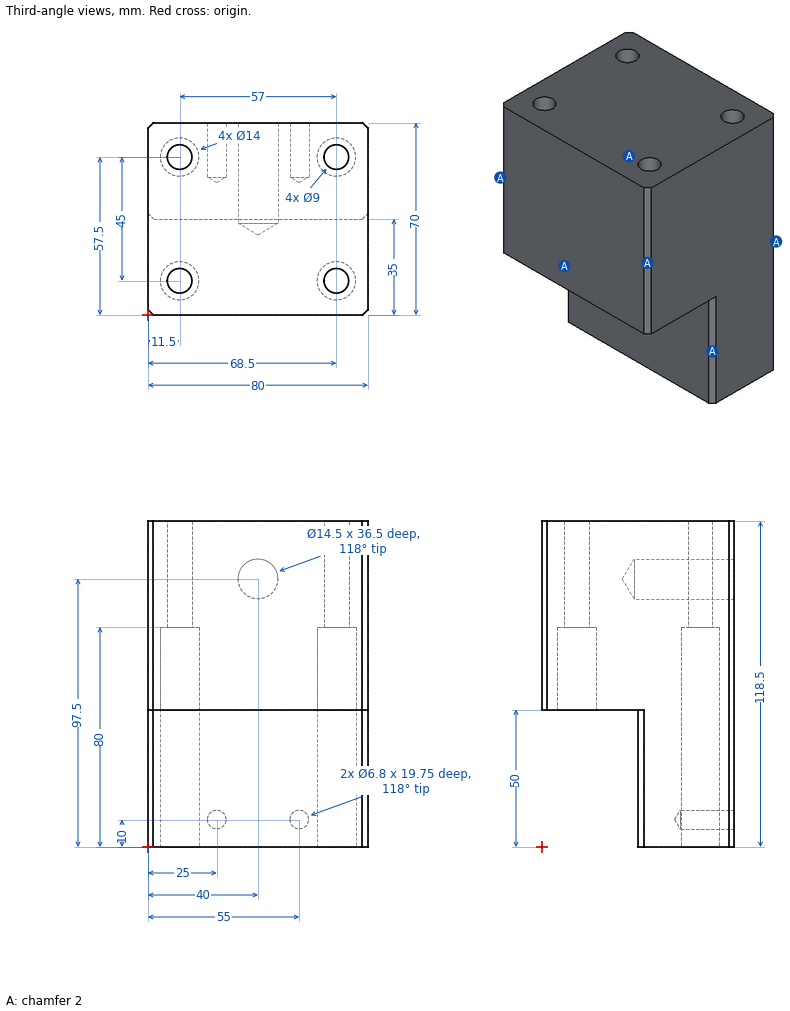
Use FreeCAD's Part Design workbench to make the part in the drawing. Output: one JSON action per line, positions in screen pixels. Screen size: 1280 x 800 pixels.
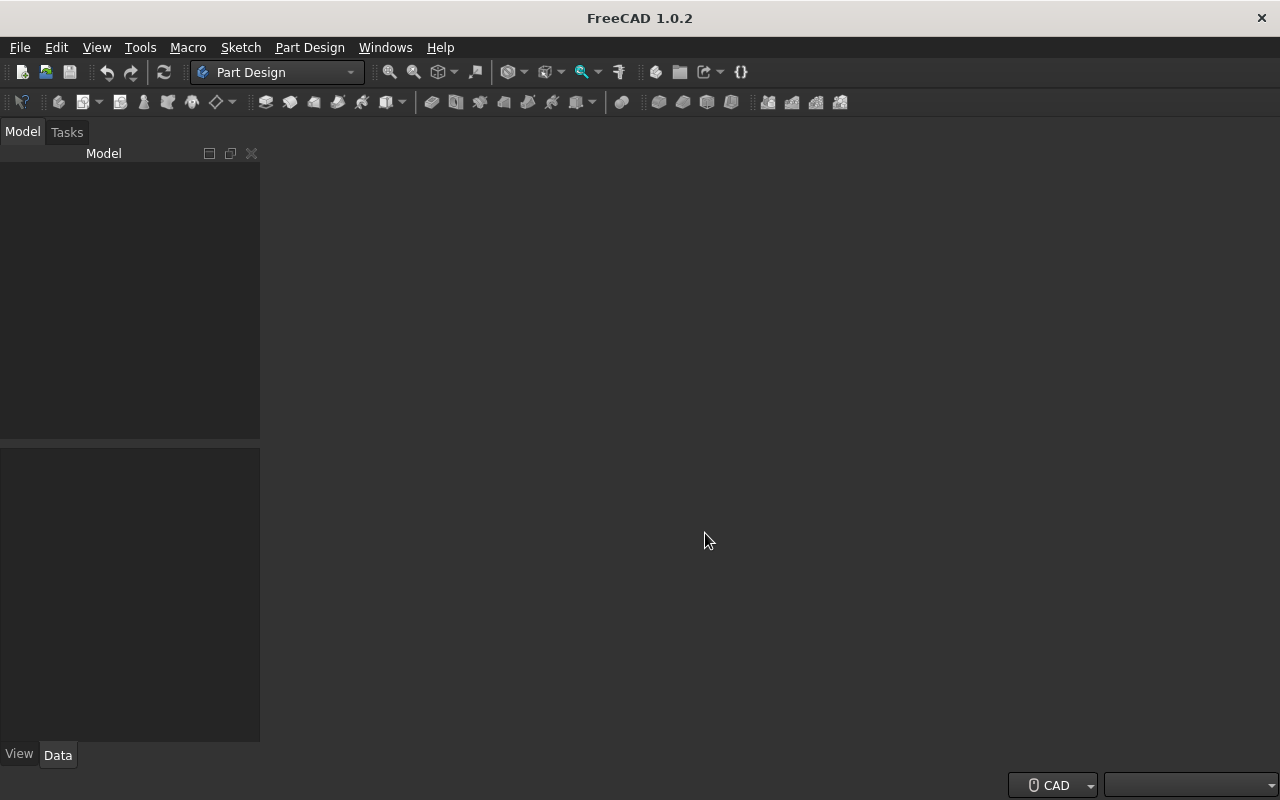
{"action": "key", "text": "ctrl+n"}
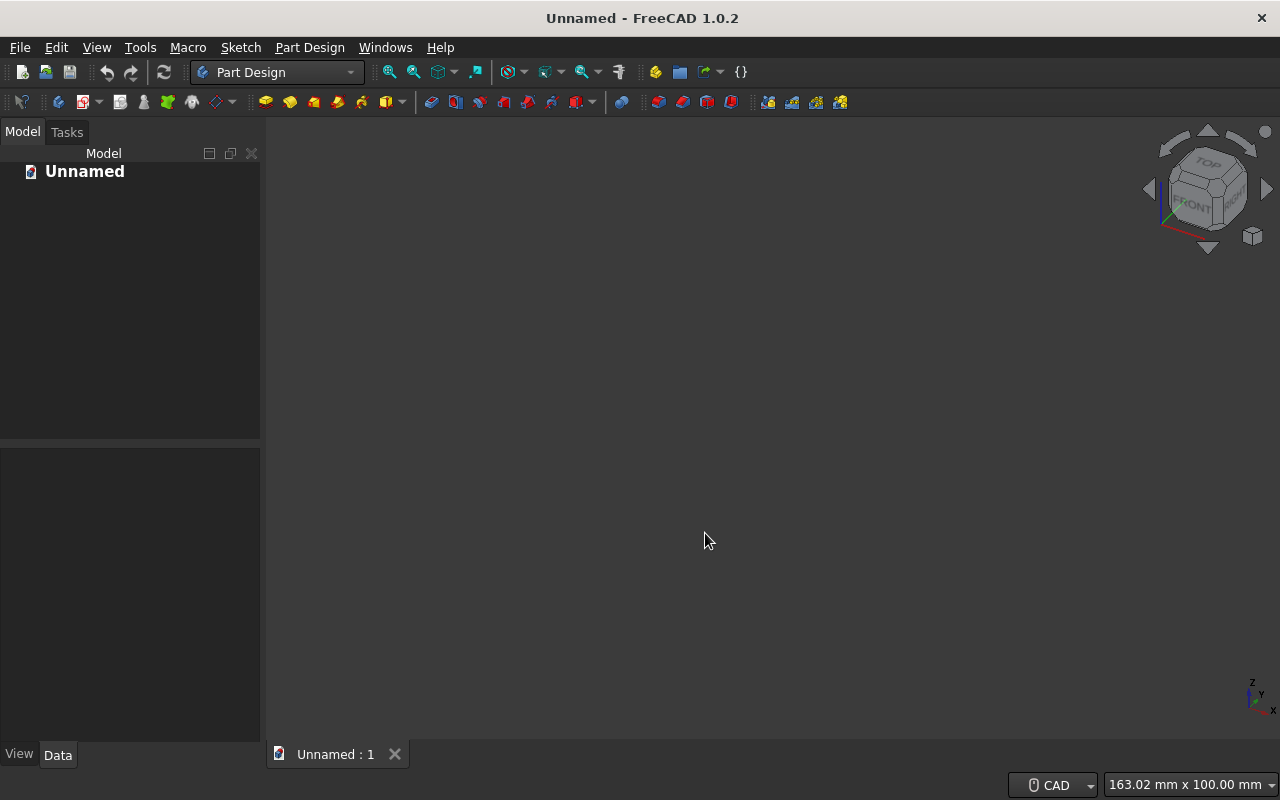
{"action": "left_click", "coordinate": [84, 102]}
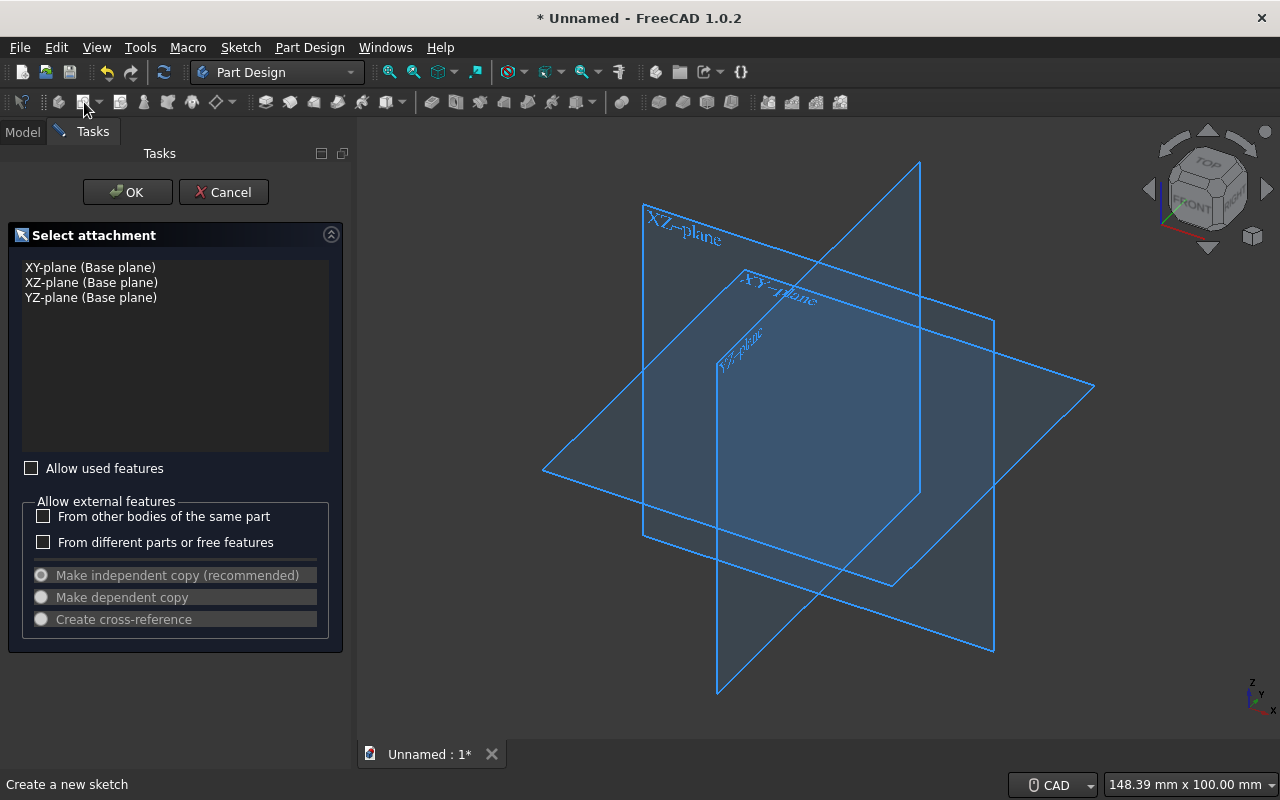
{"action": "left_click", "coordinate": [82, 268]}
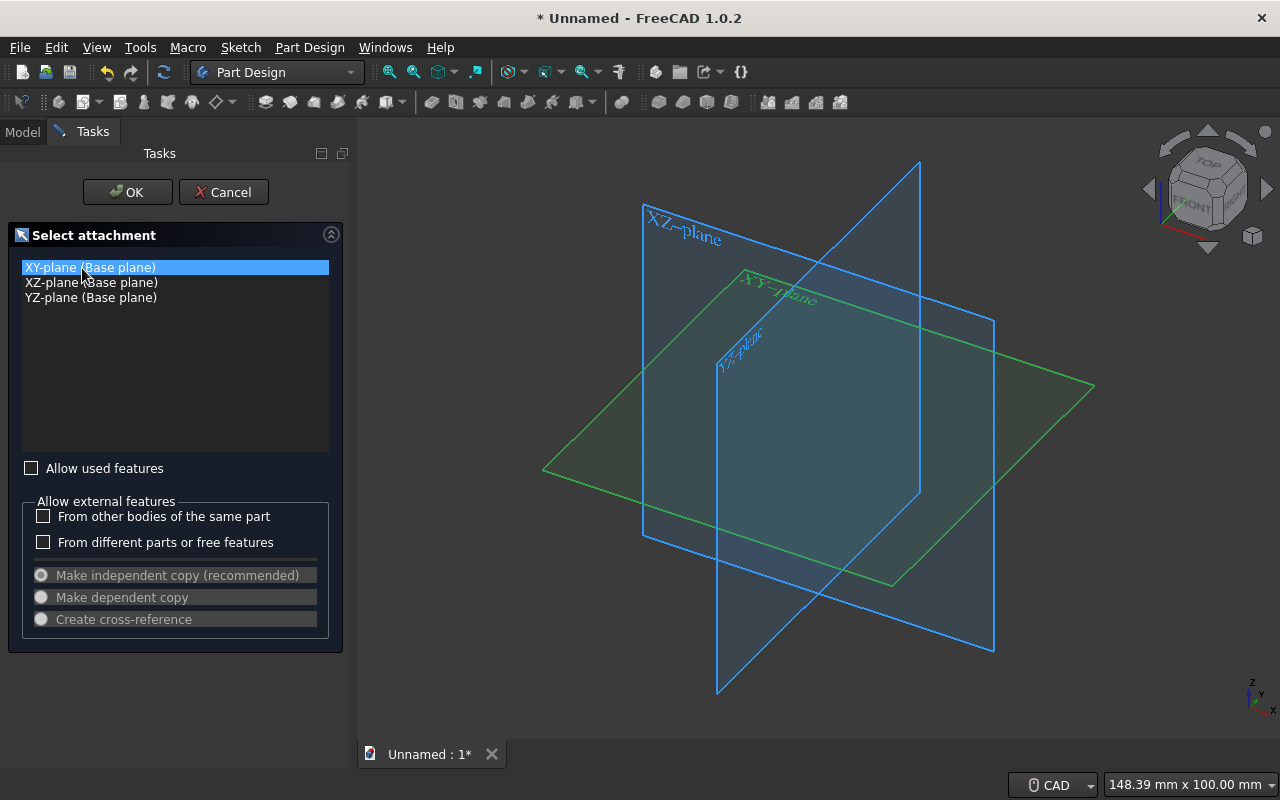
{"action": "left_click", "coordinate": [128, 192]}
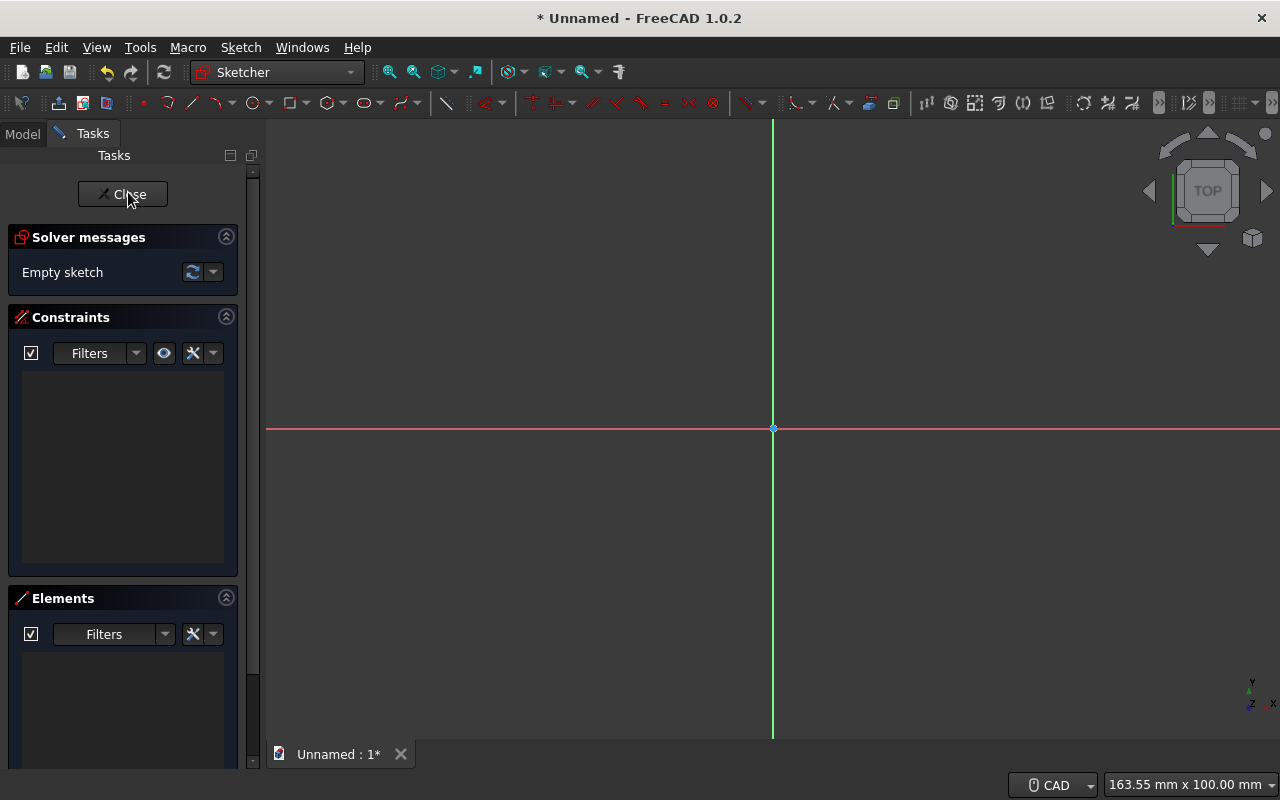
{"action": "scroll", "coordinate": [294, 711], "scroll_direction": "down", "scroll_amount": 2}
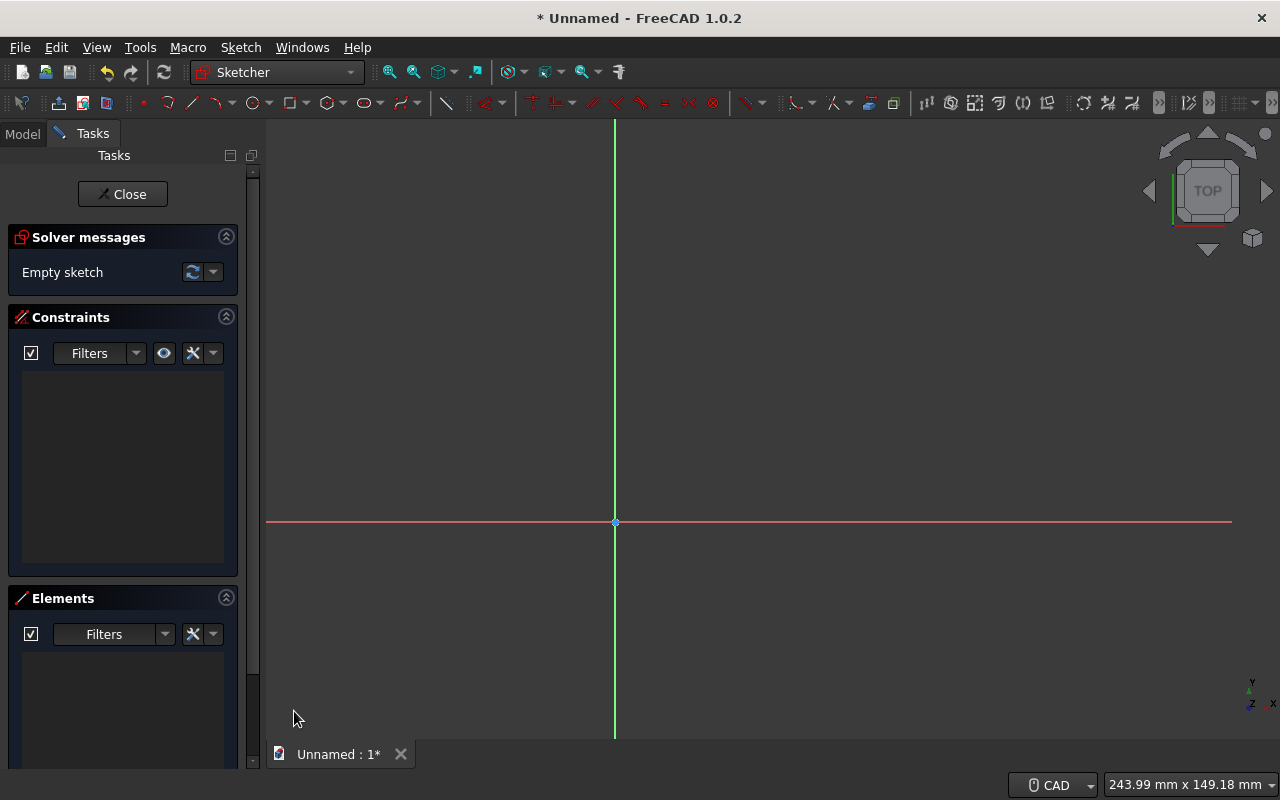
{"action": "scroll", "coordinate": [938, 271], "scroll_direction": "up", "scroll_amount": 2}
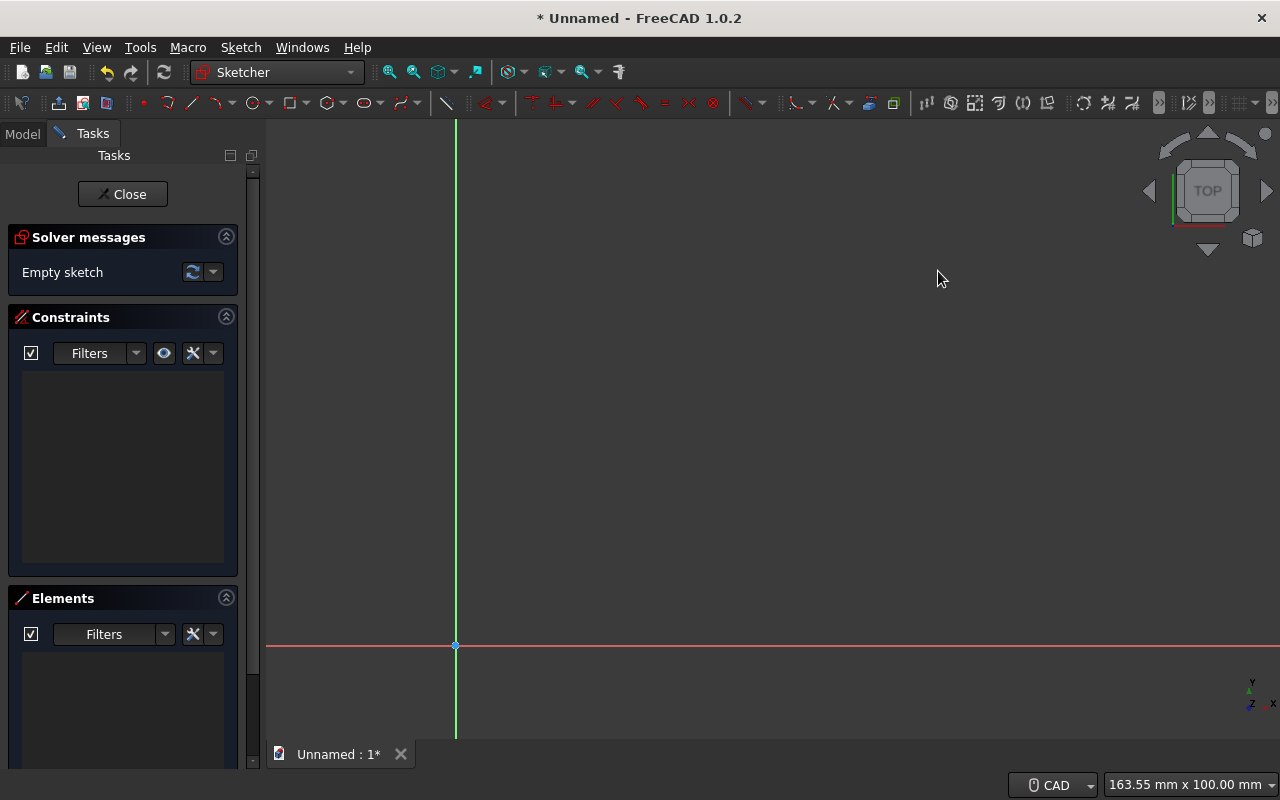
{"action": "key", "text": "g r"}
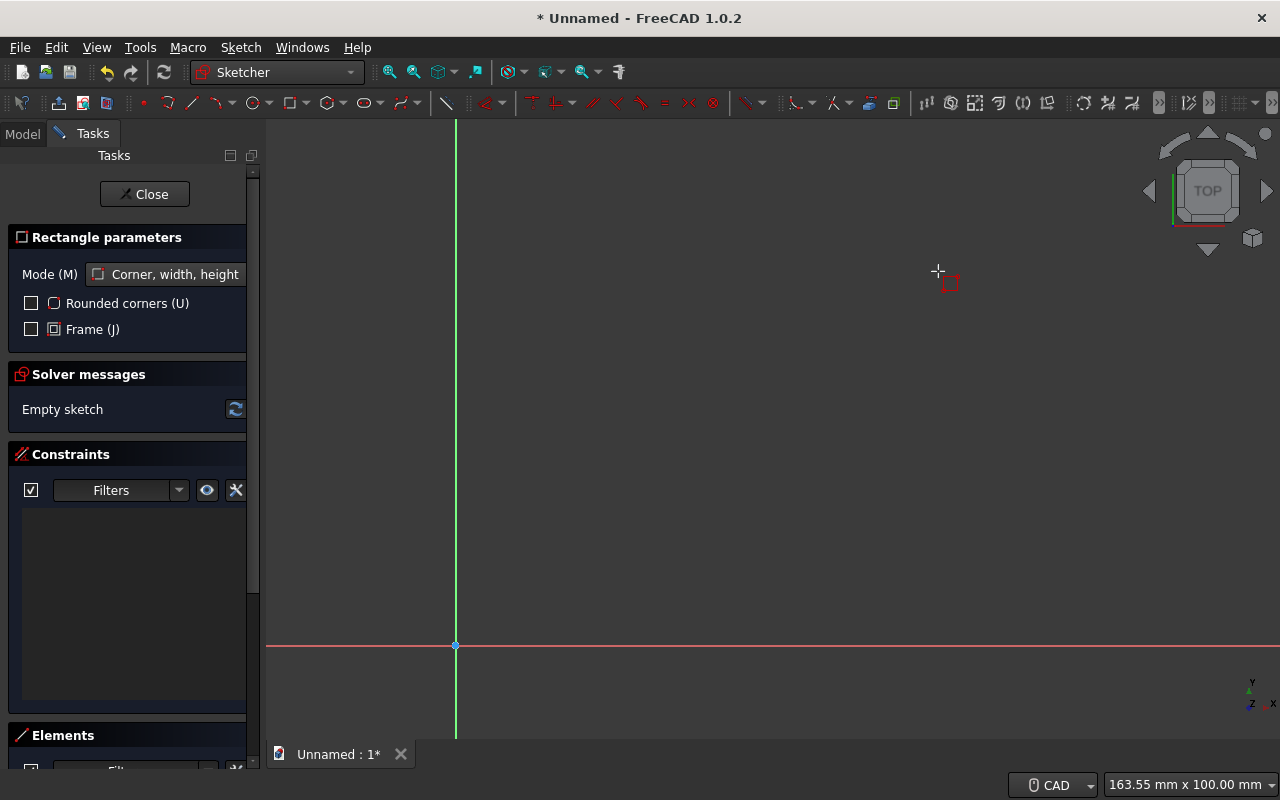
{"action": "left_click", "coordinate": [456, 646]}
{"action": "left_click", "coordinate": [952, 212]}
{"action": "key", "text": "Escape"}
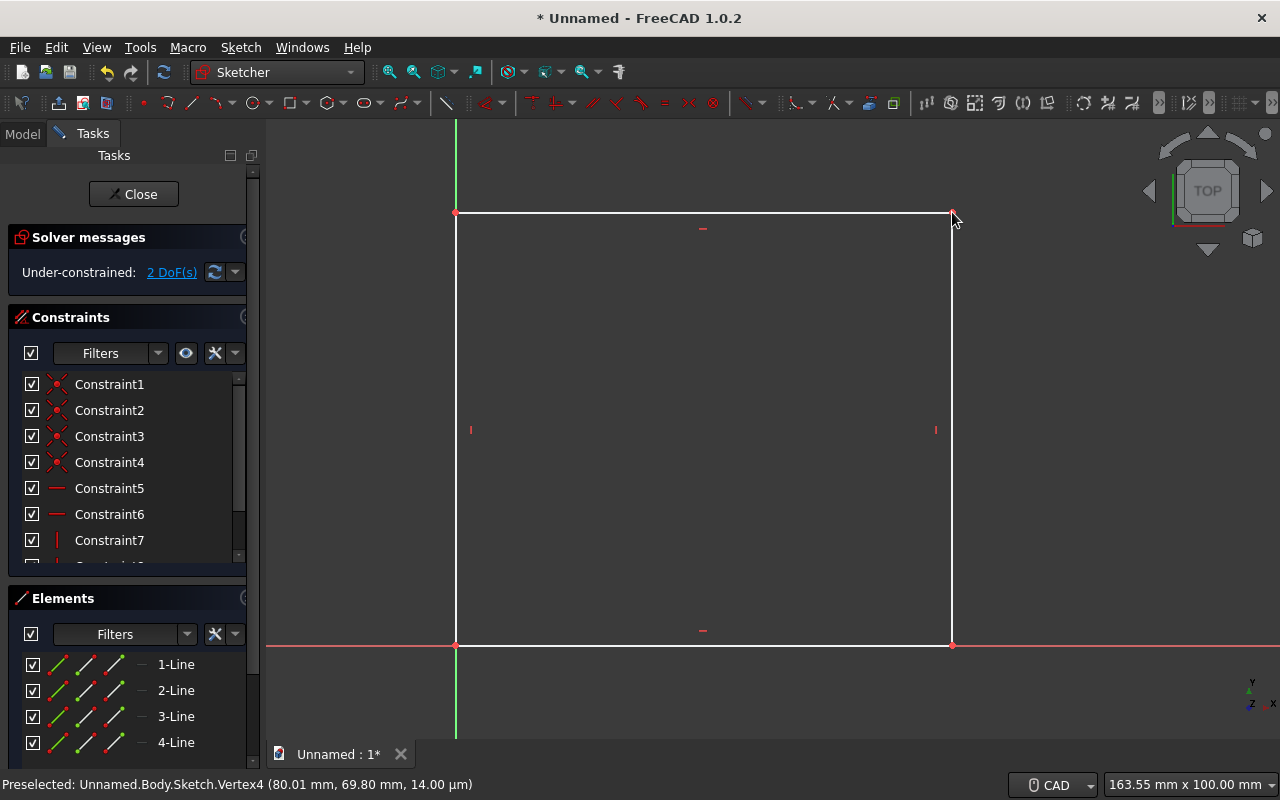
{"action": "left_click", "coordinate": [486, 104]}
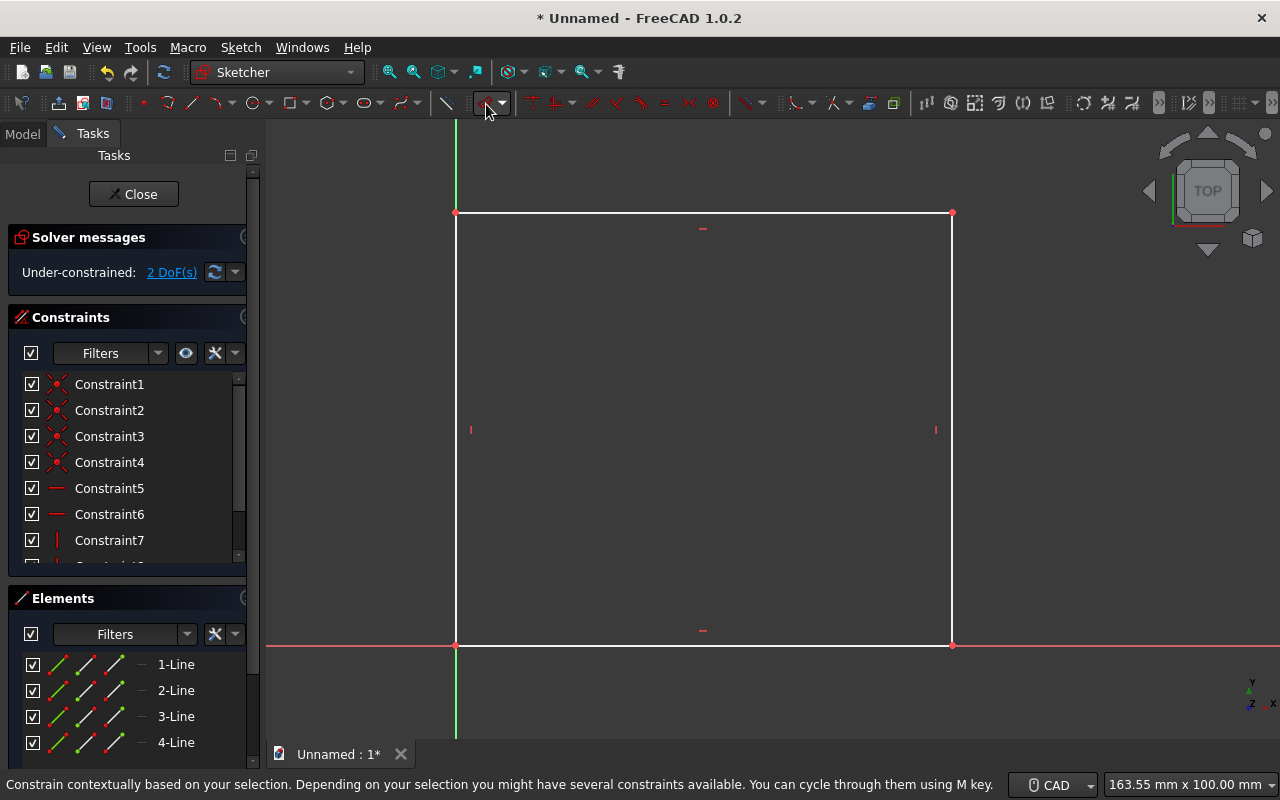
{"action": "left_click", "coordinate": [605, 646]}
{"action": "left_click", "coordinate": [704, 680]}